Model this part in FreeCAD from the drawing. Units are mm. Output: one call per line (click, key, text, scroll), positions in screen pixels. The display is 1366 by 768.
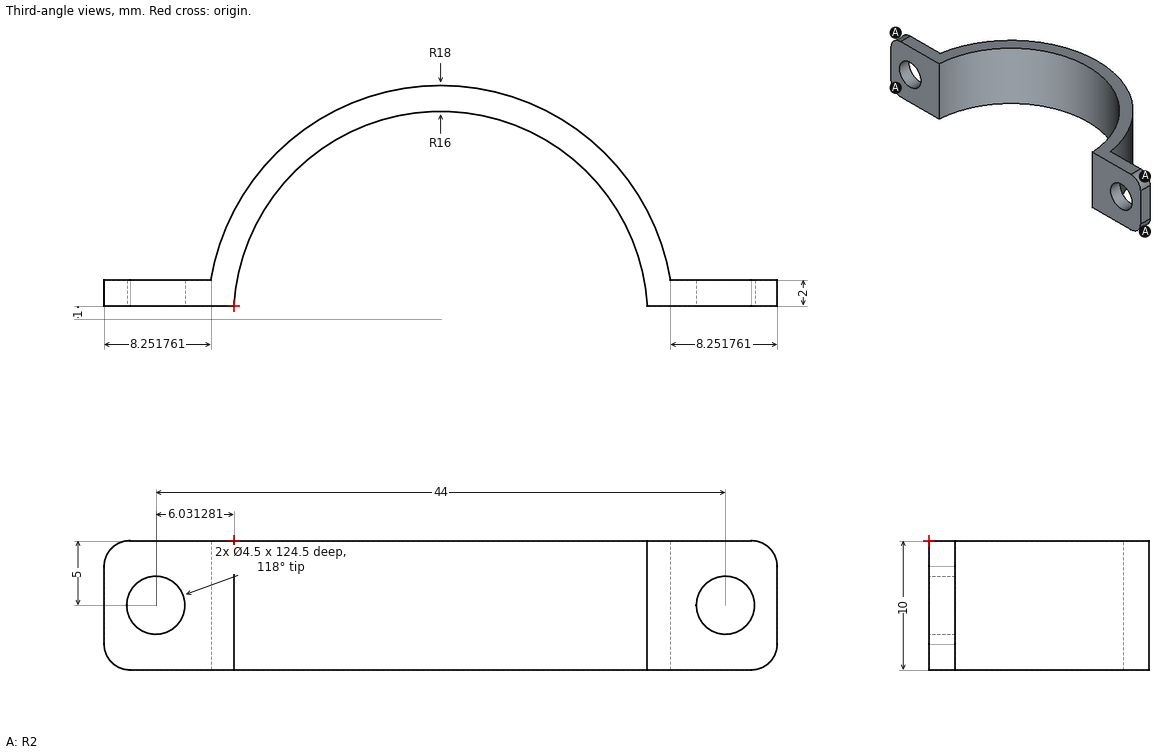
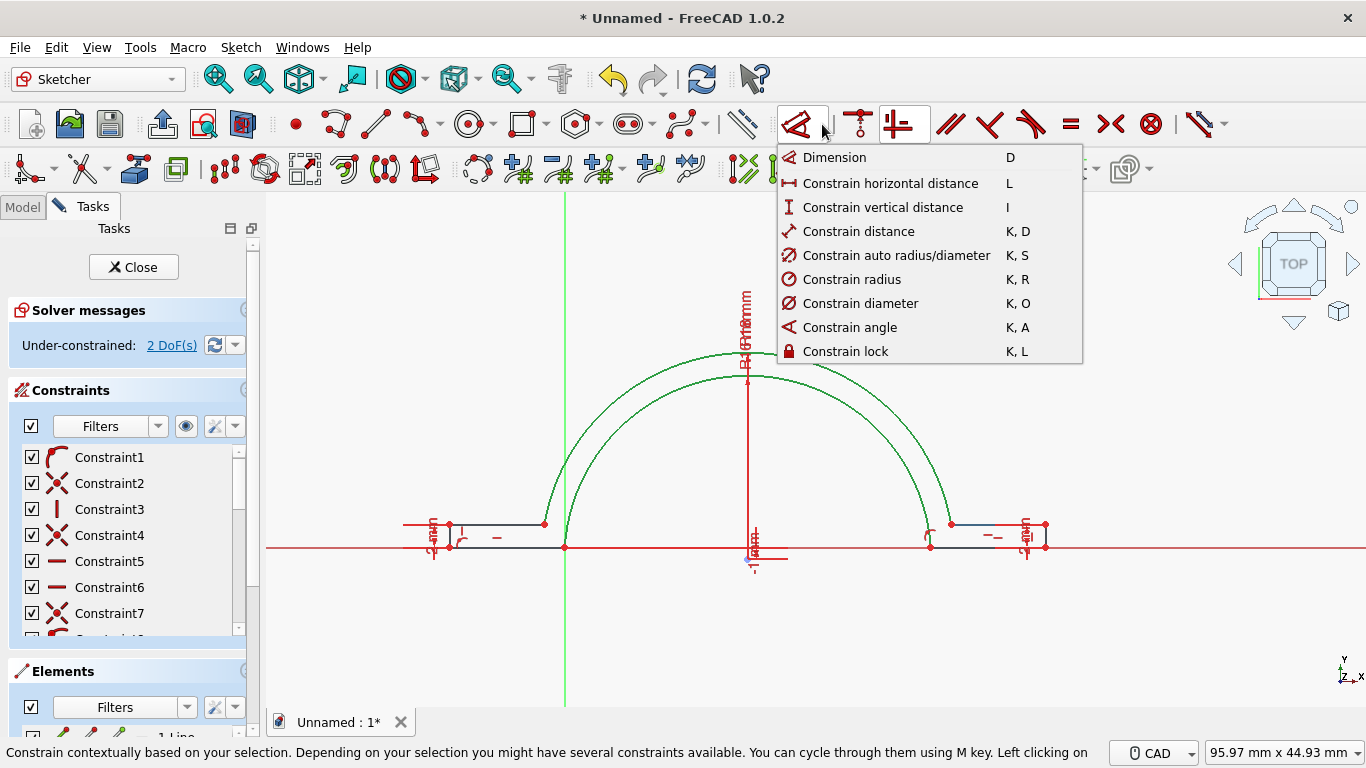
click(930, 183)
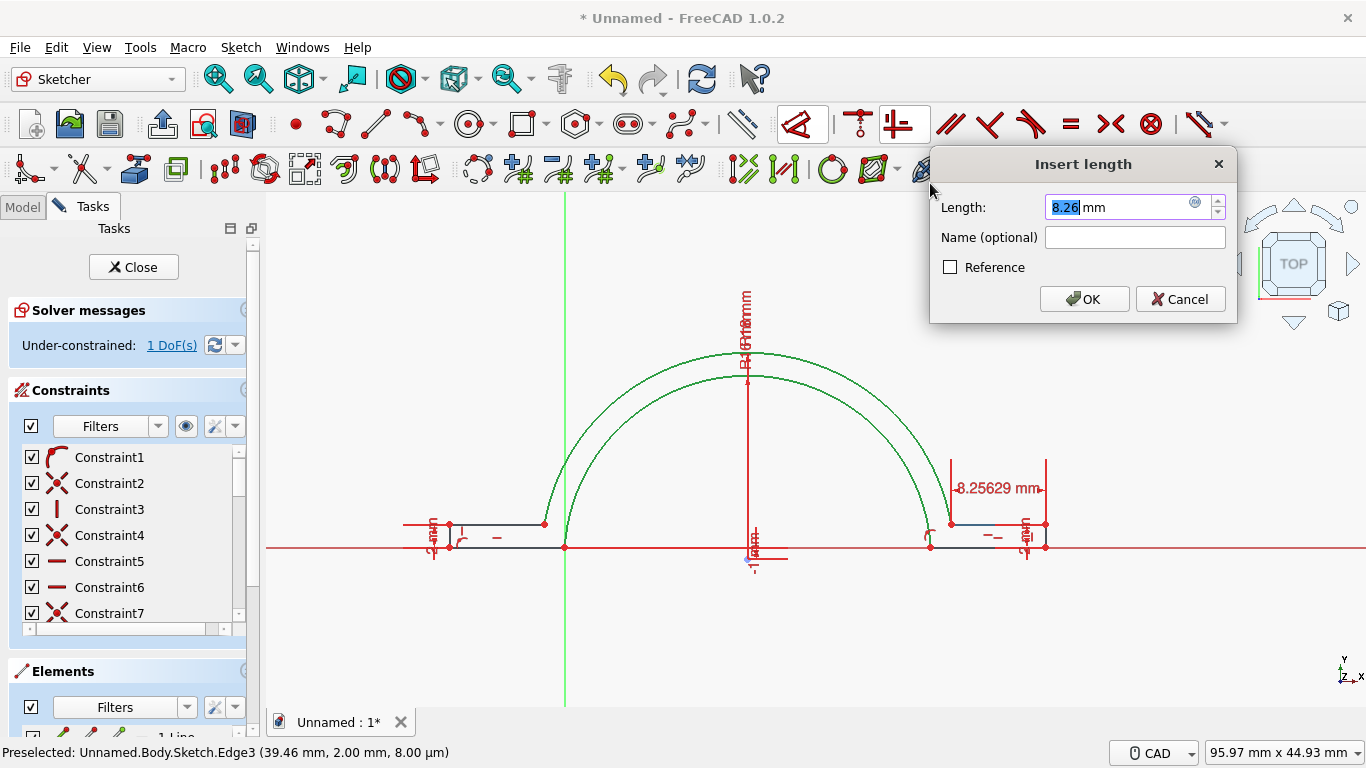
text(8.251761)
key(Return)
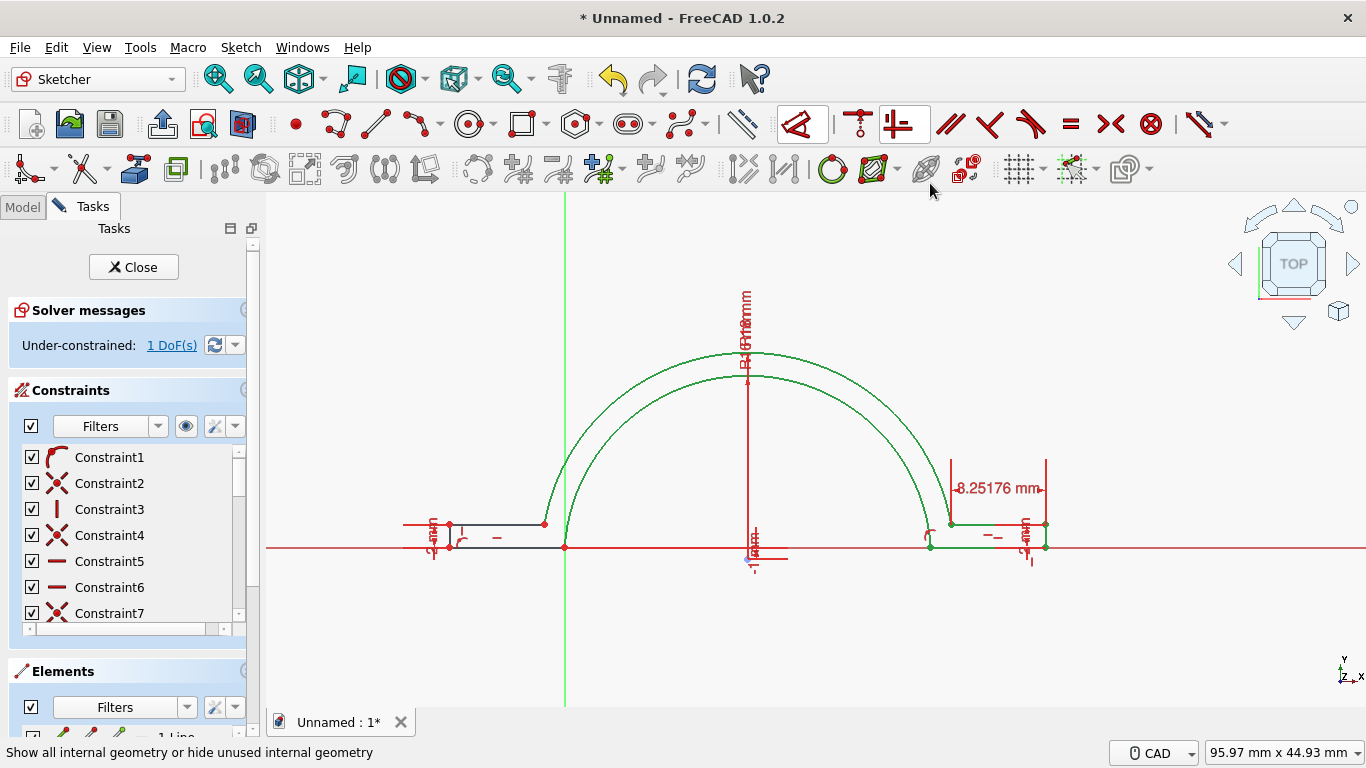
click(516, 525)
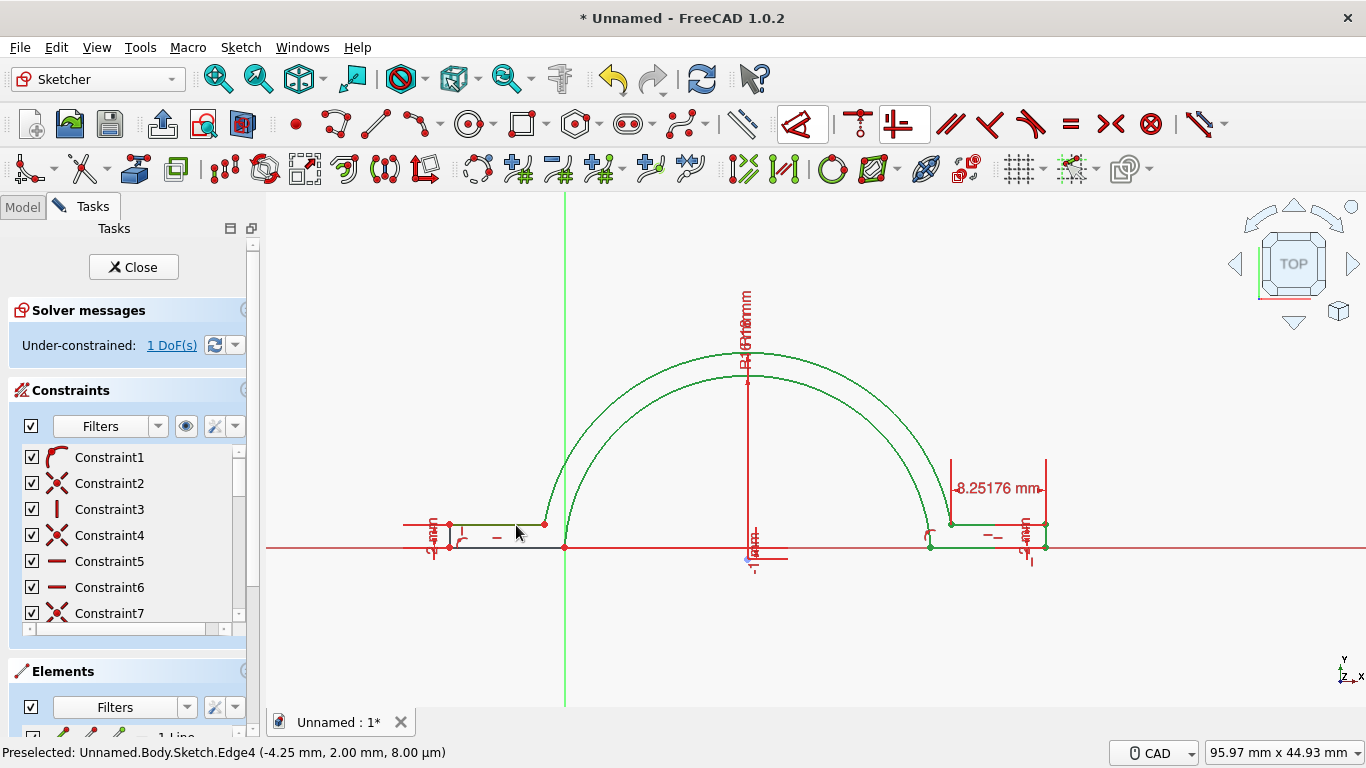
key(l)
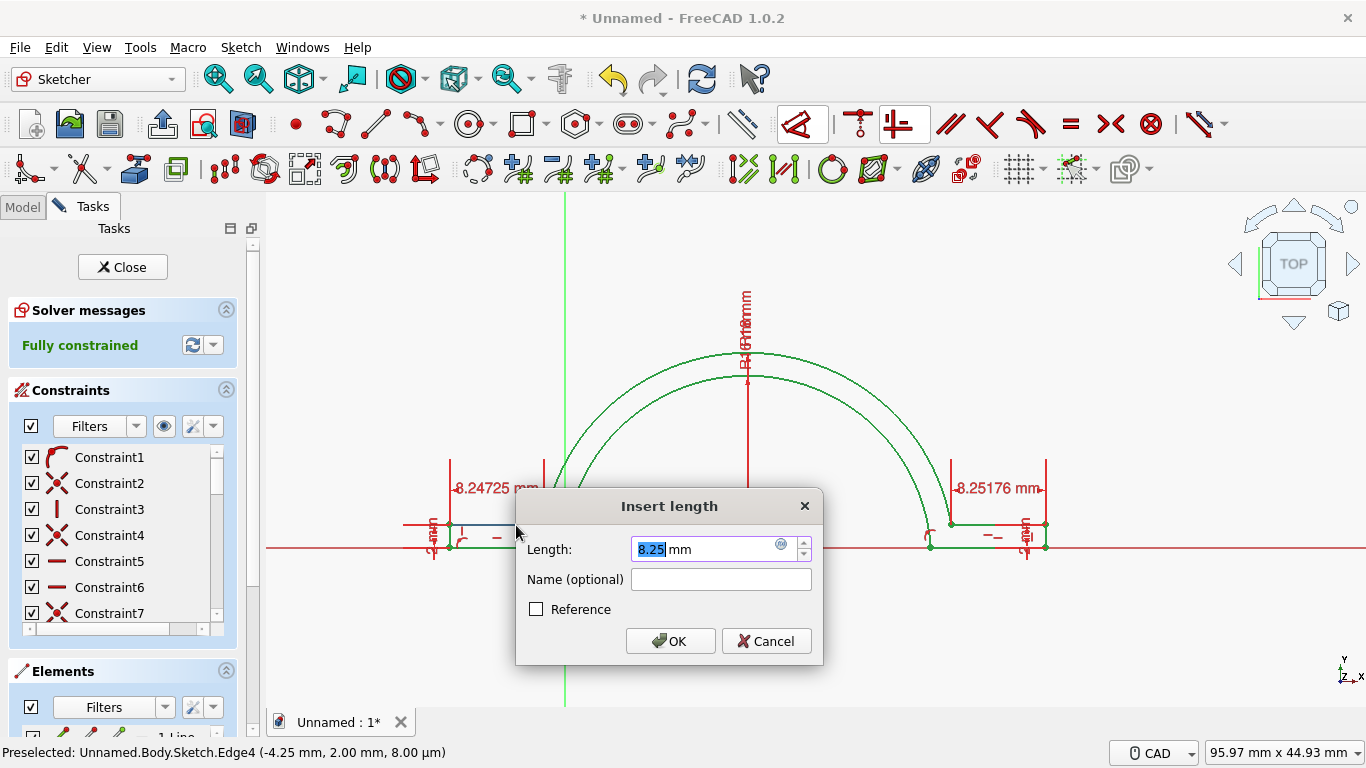
text(8.251761)
key(Return)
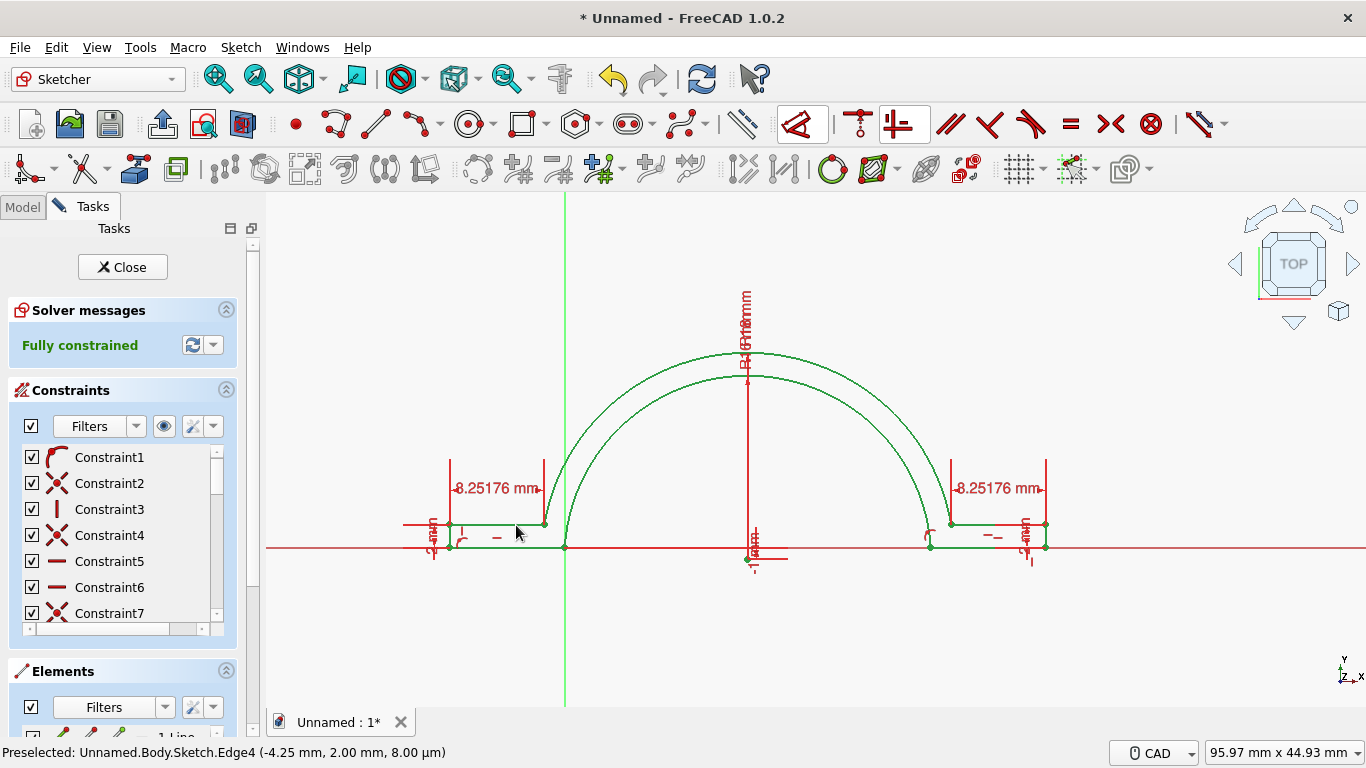
click(123, 267)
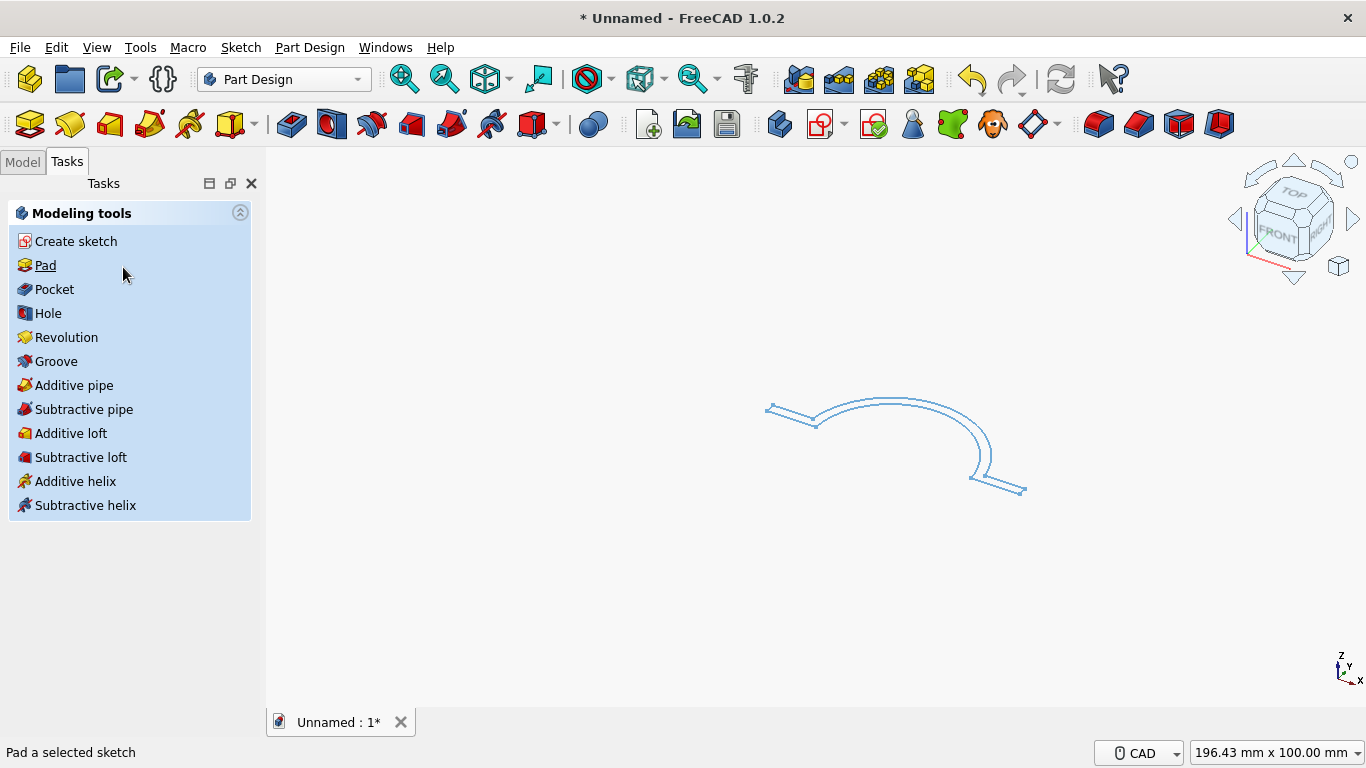
click(30, 124)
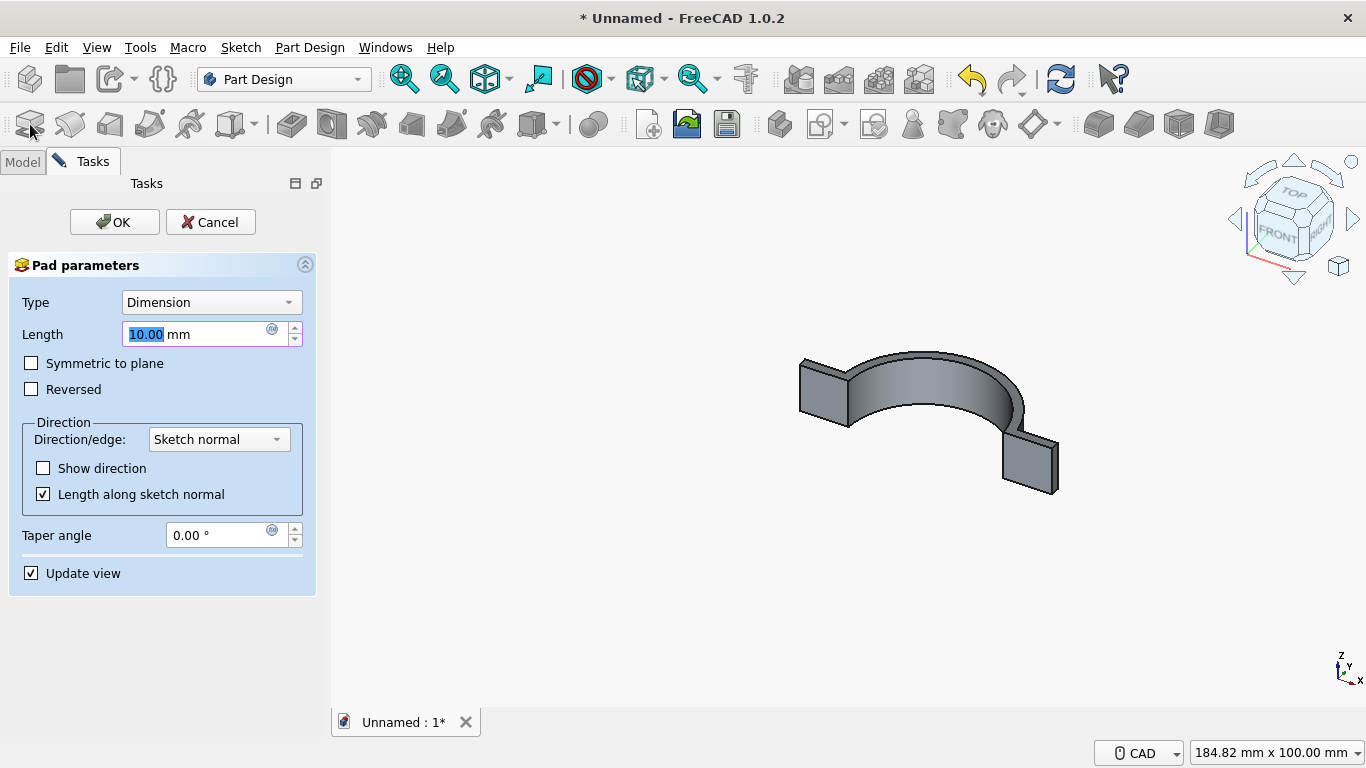
text(10)
key(Tab)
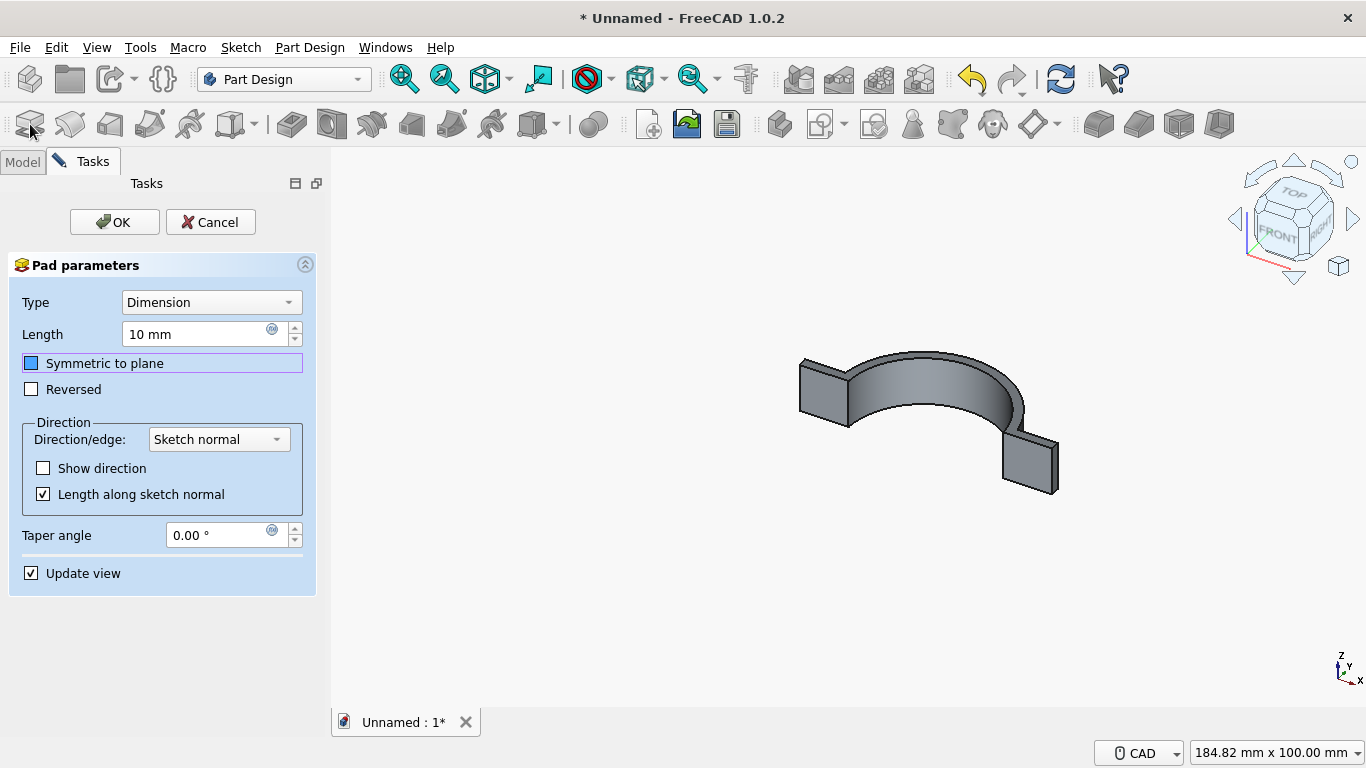
click(30, 389)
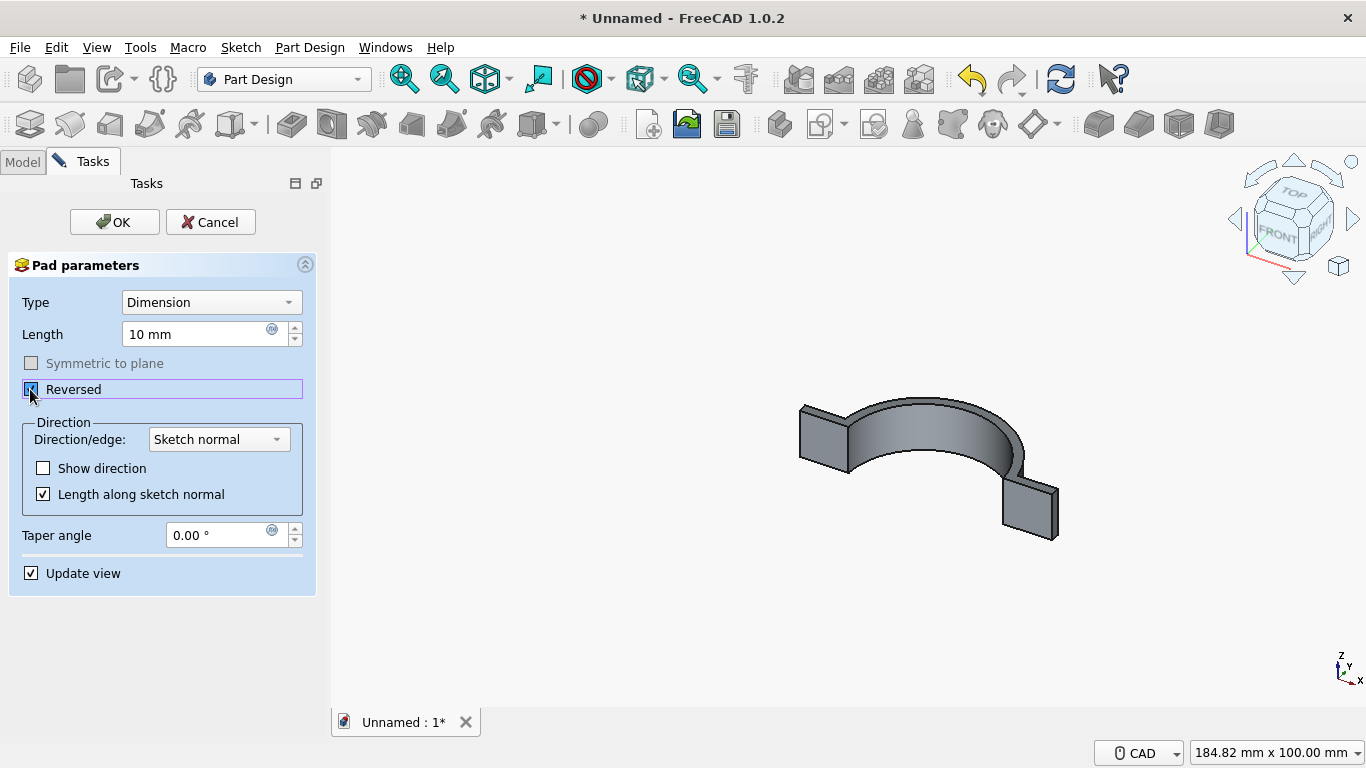
click(115, 222)